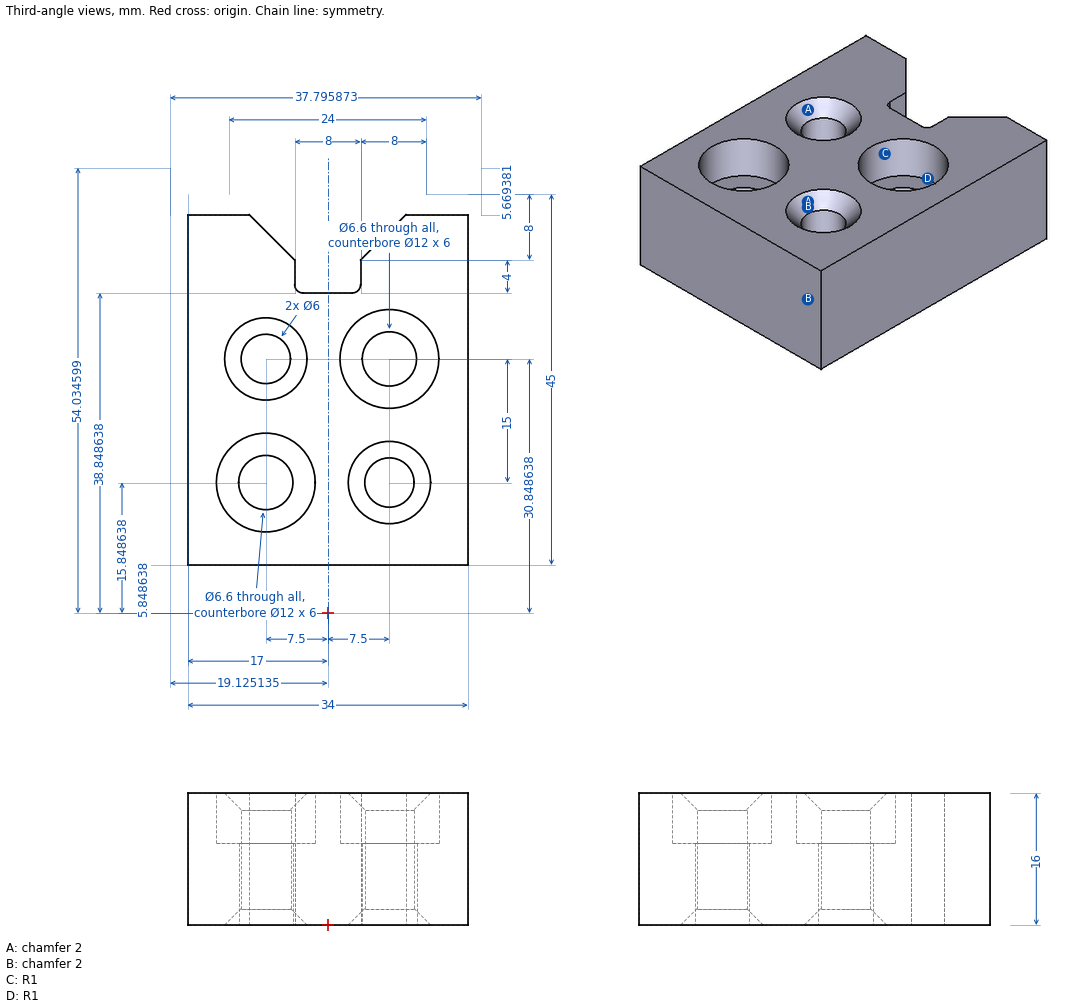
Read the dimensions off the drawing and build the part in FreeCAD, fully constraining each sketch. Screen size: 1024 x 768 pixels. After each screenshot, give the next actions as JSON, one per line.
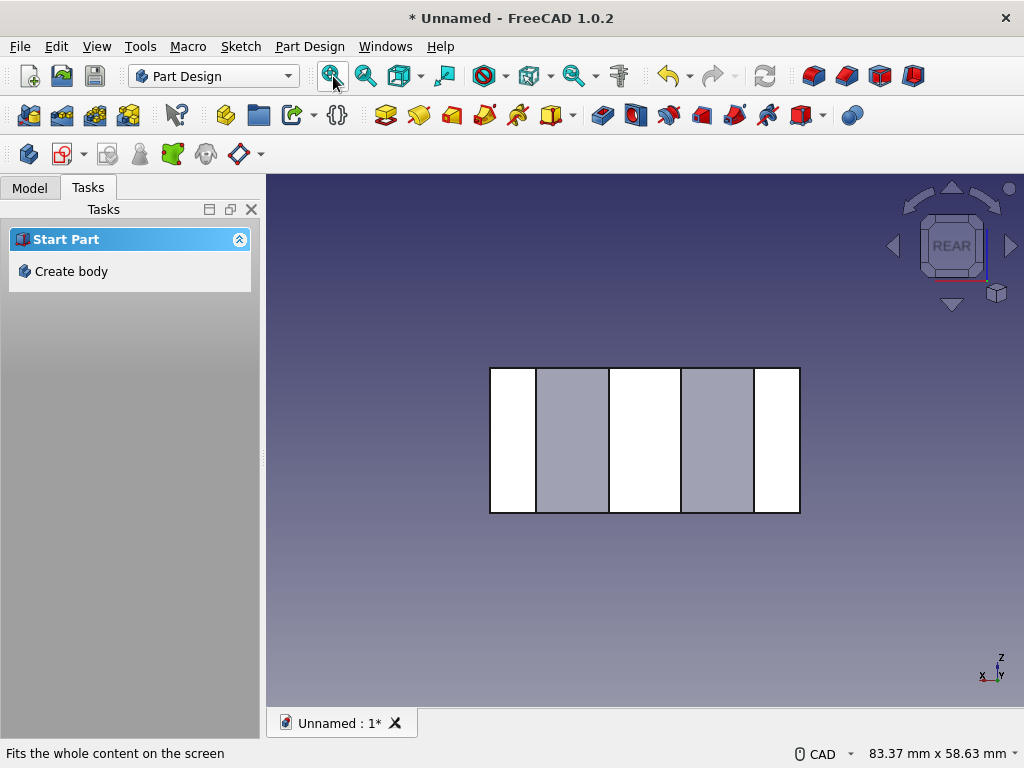
{"action": "left_click", "coordinate": [333, 76]}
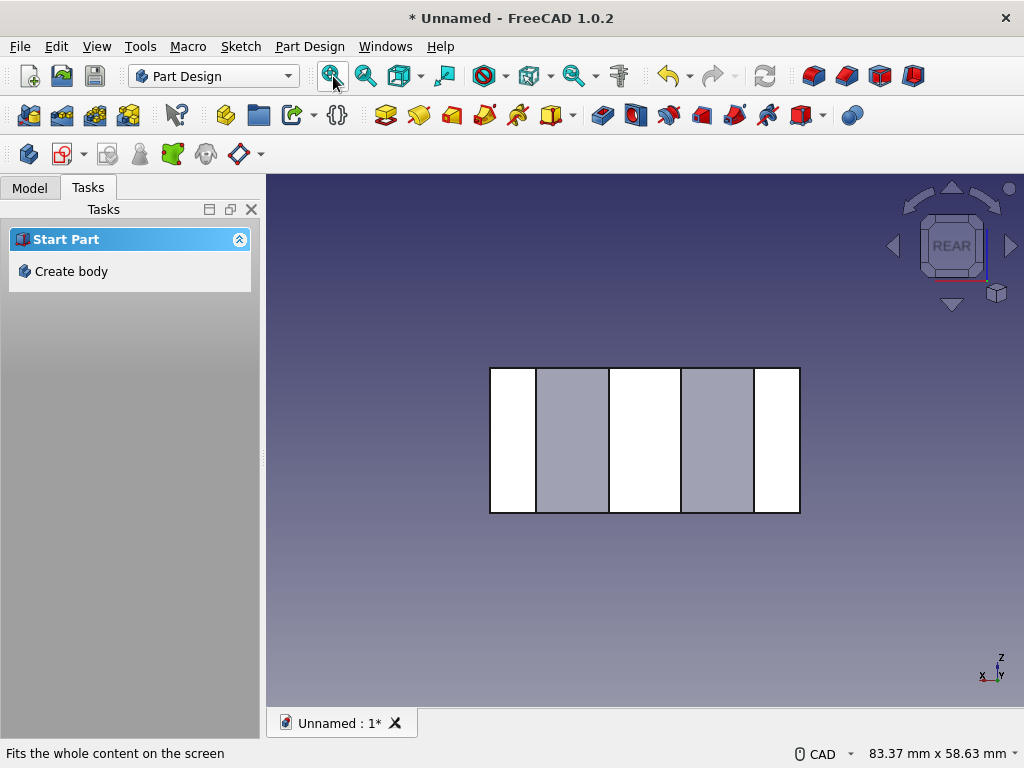
{"action": "key", "text": "6"}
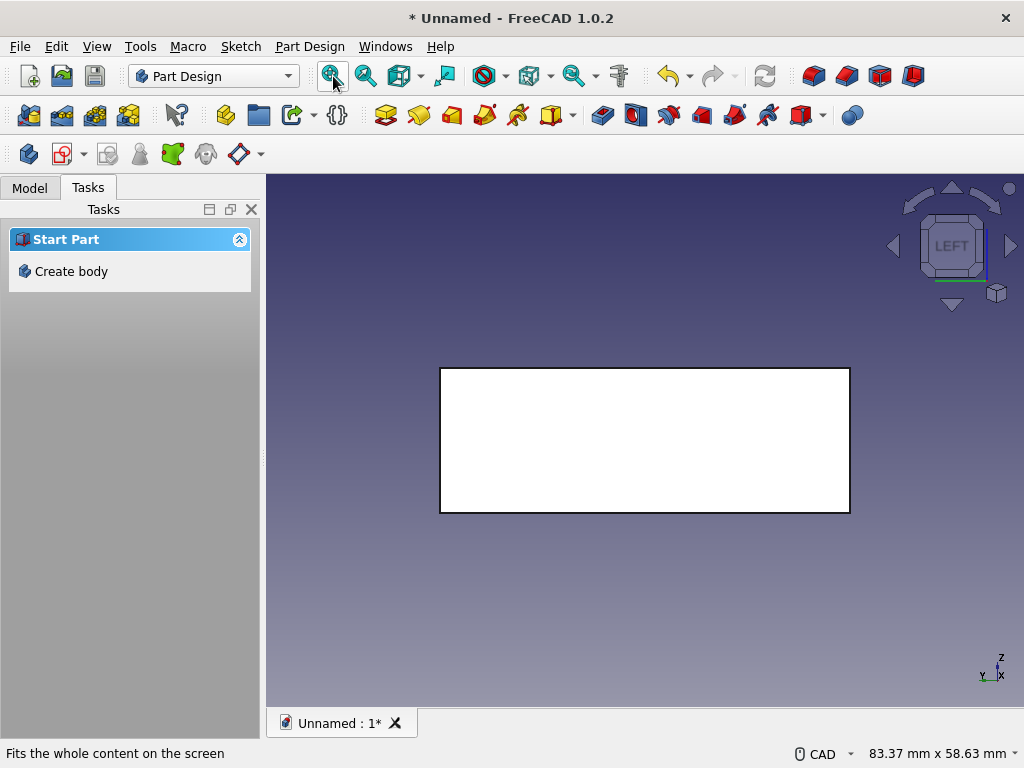
{"action": "key", "text": "v 3"}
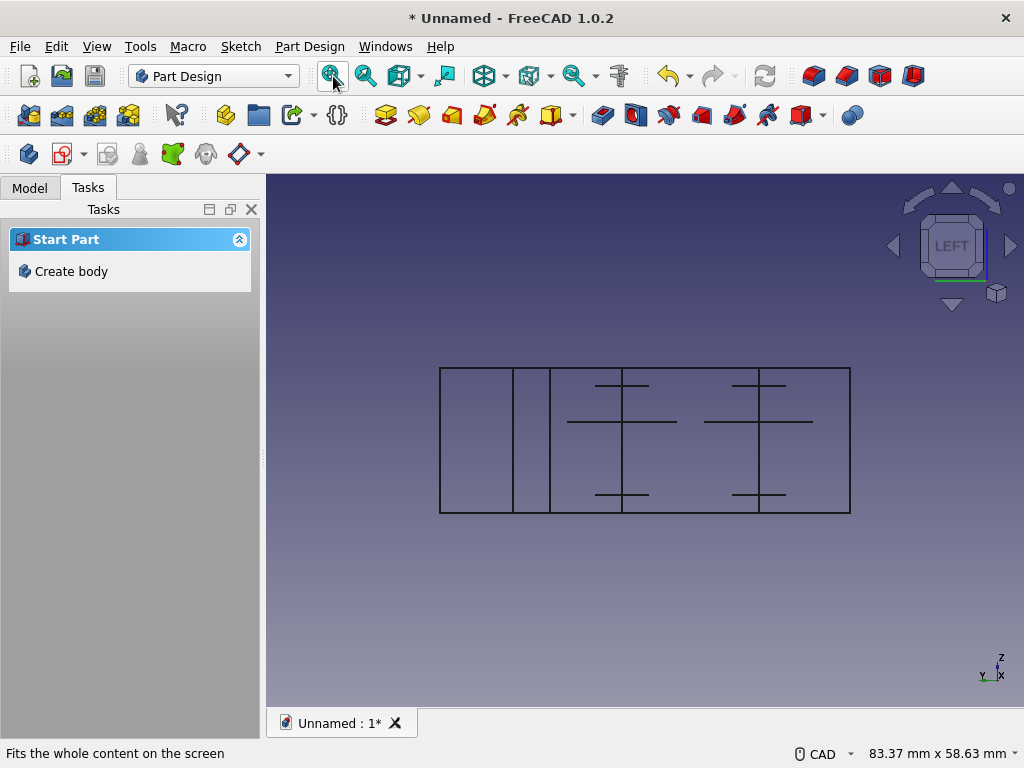
{"action": "key", "text": "0"}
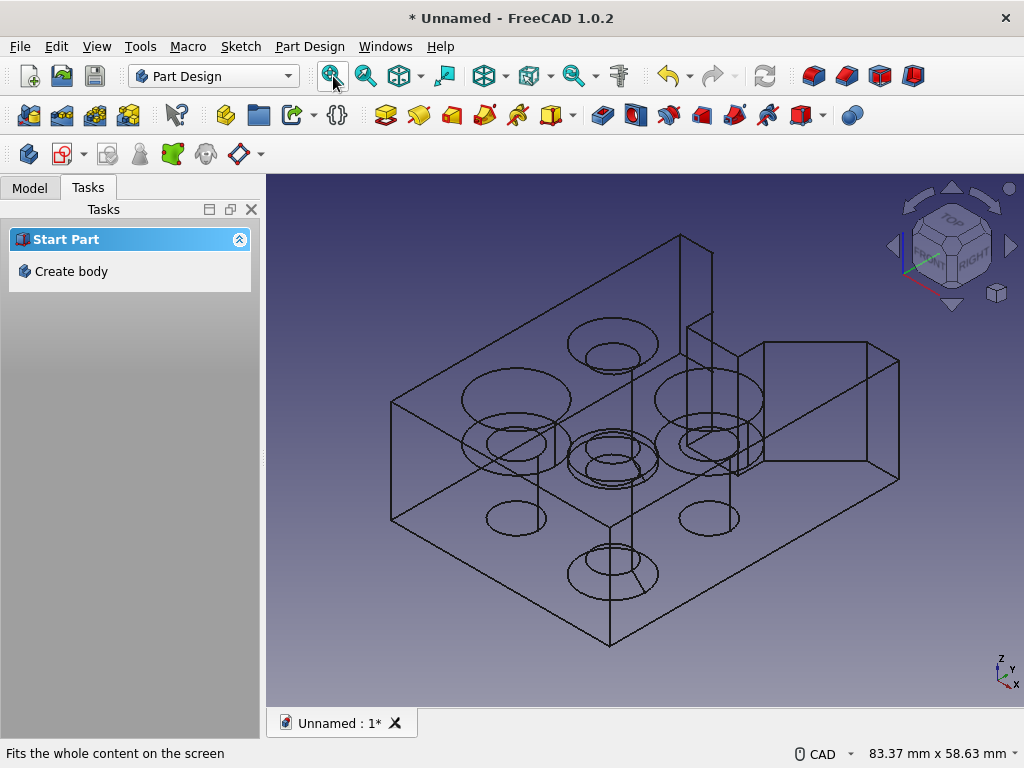
{"action": "left_click", "coordinate": [687, 386]}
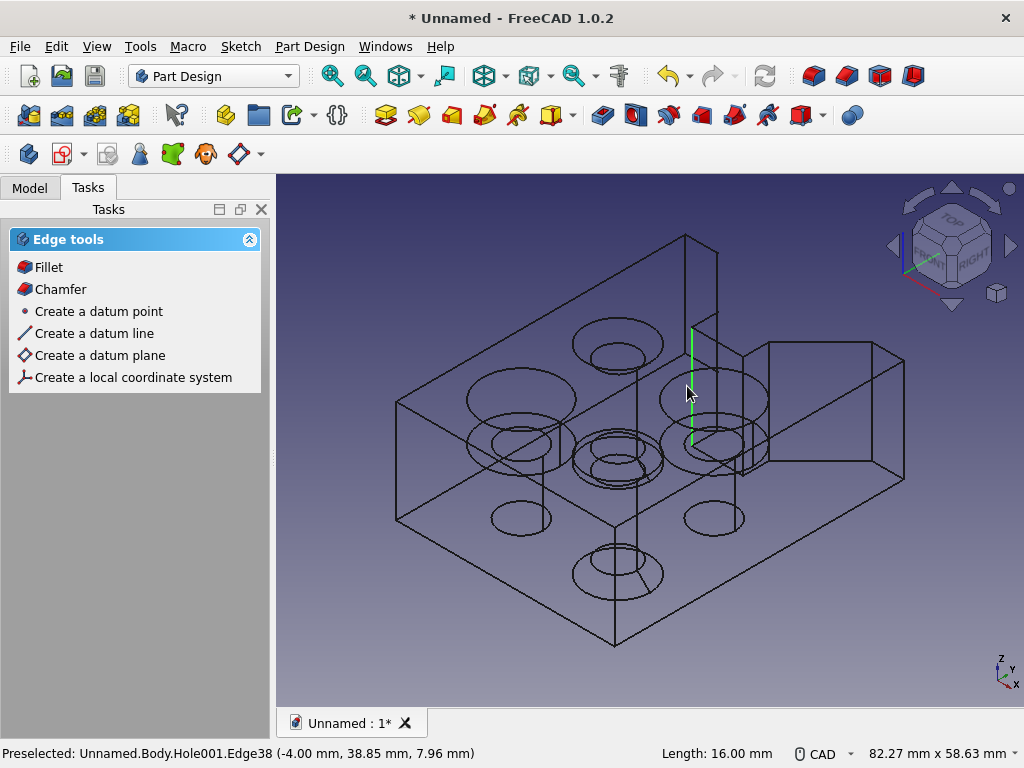
{"action": "key", "text": "v 1"}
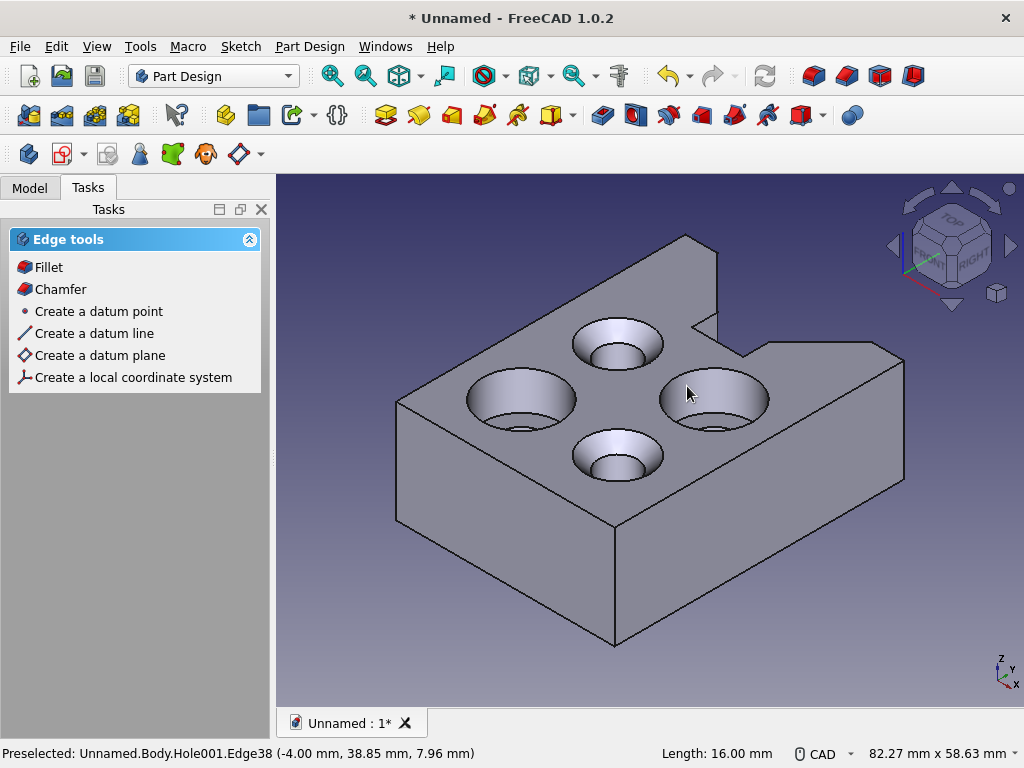
{"action": "left_click", "coordinate": [814, 76]}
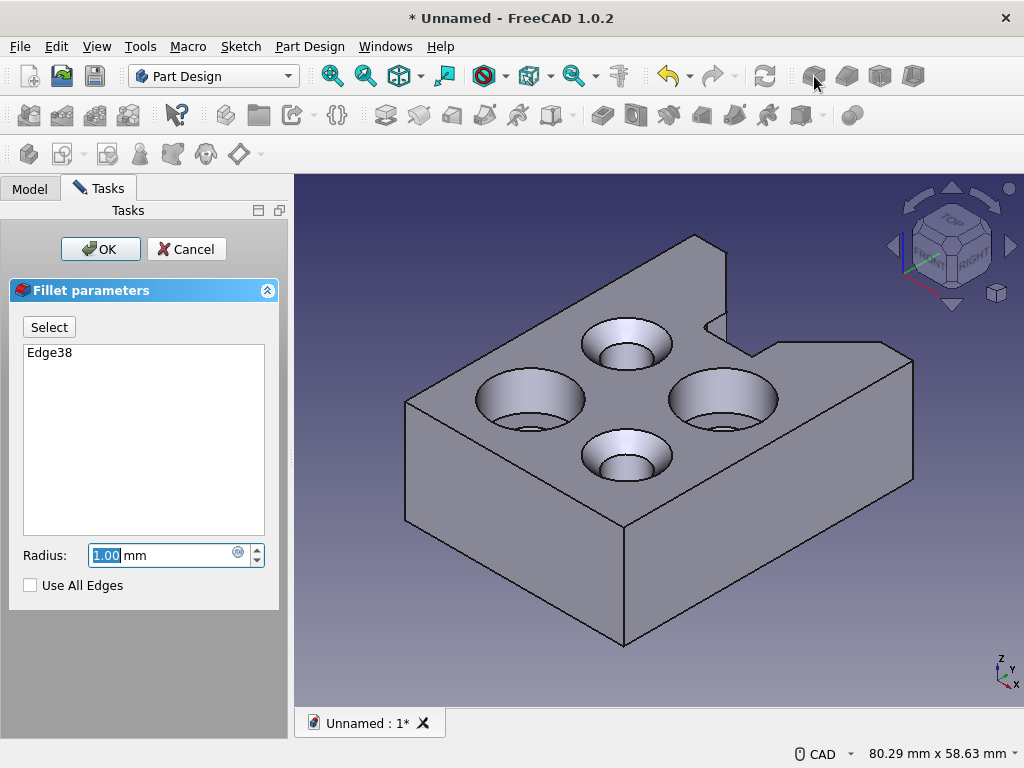
{"action": "type", "text": "1"}
{"action": "key", "text": "Tab"}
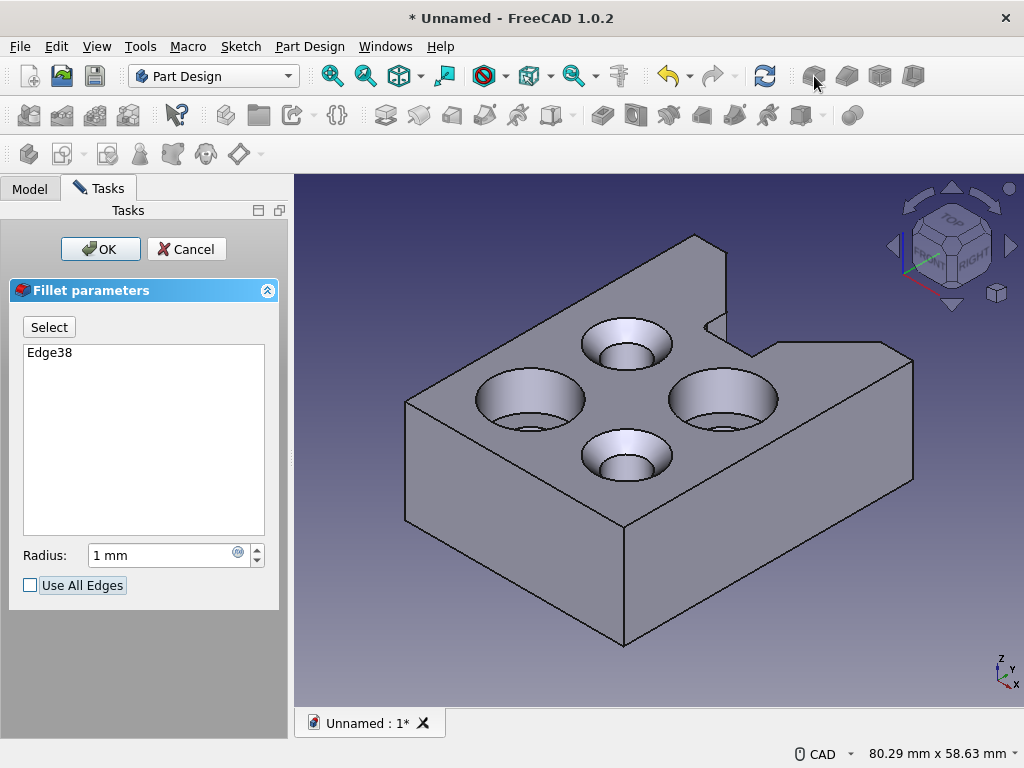
{"action": "left_click", "coordinate": [101, 249]}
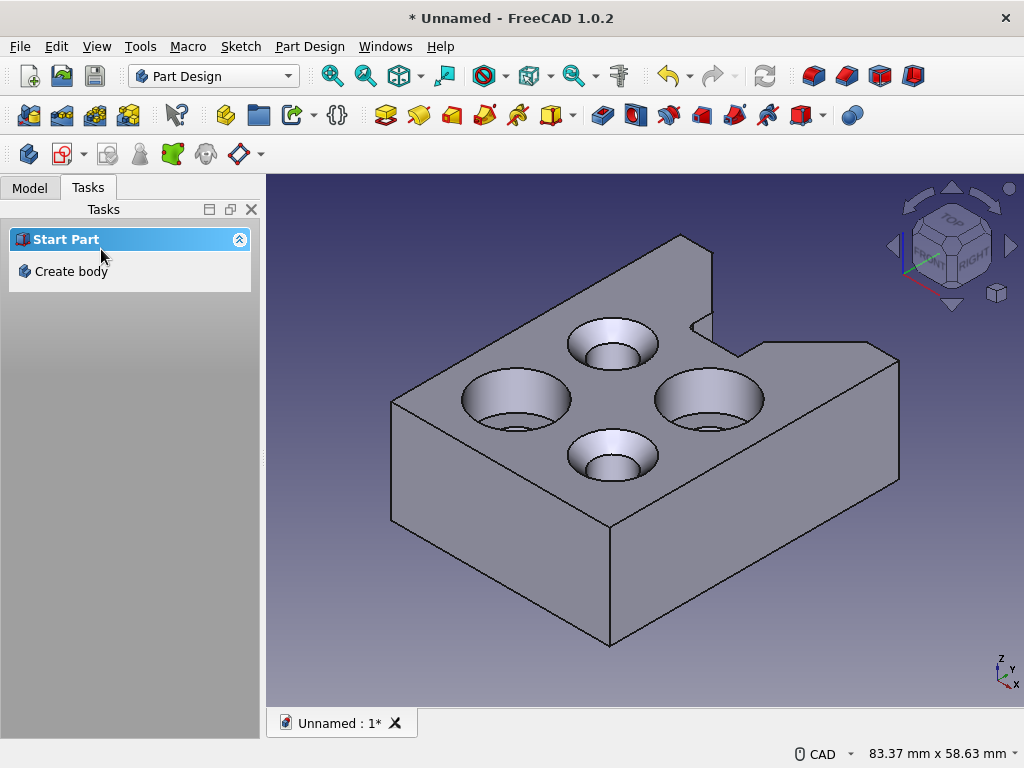
{"action": "key", "text": "2"}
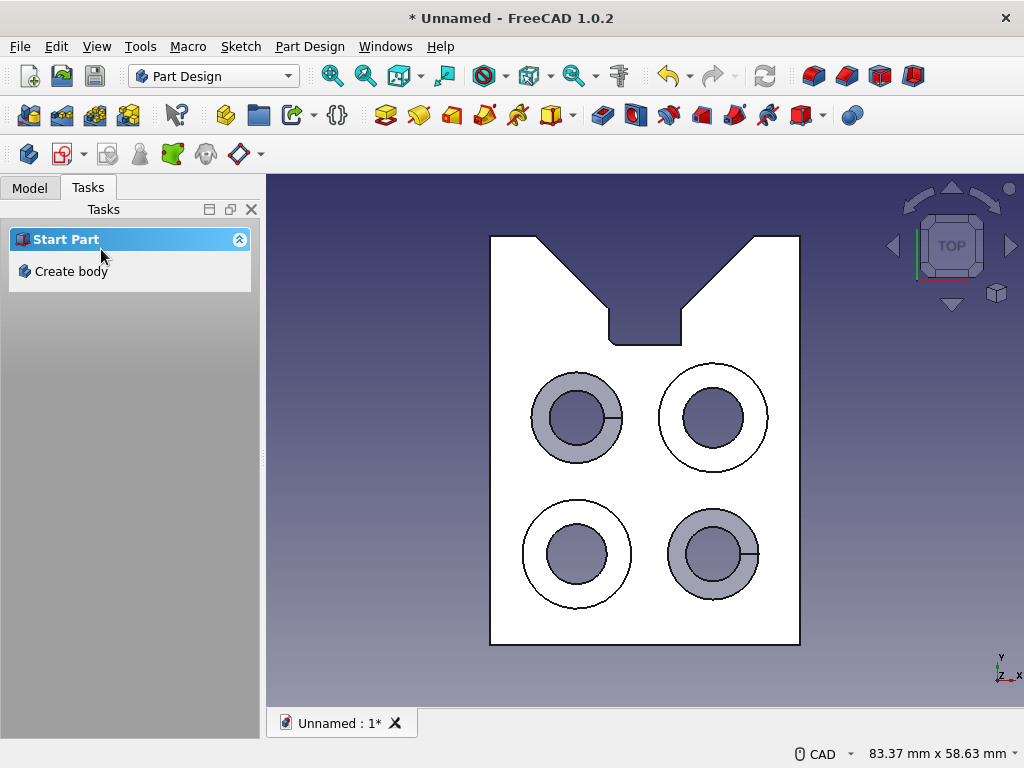
{"action": "key", "text": "0"}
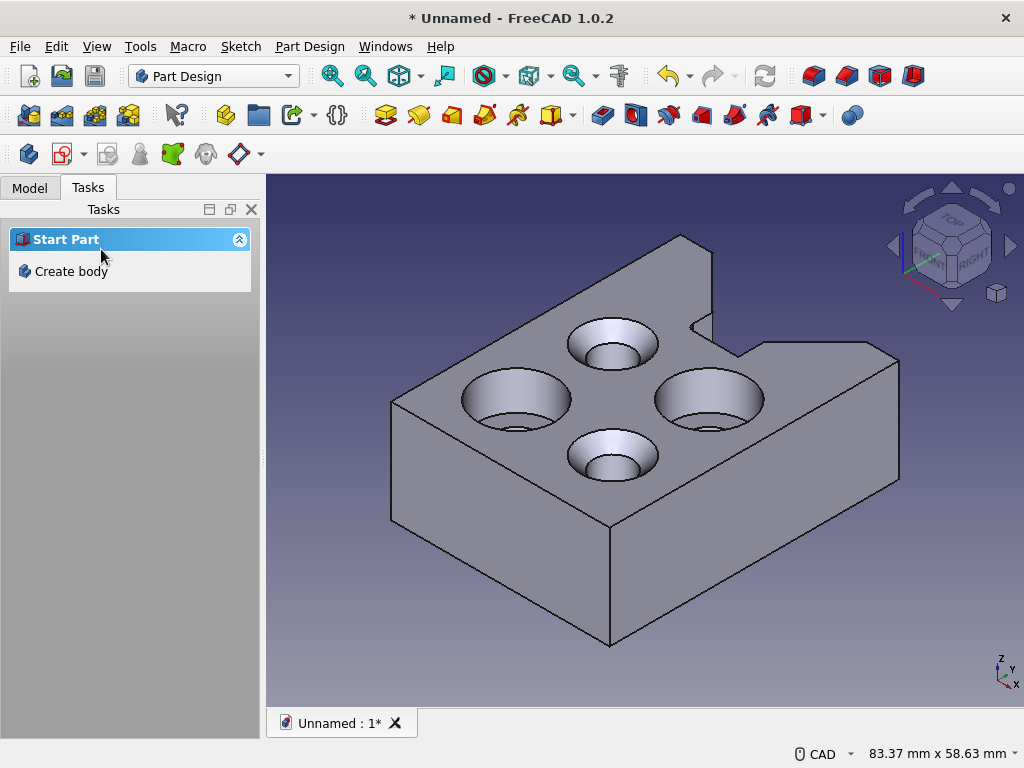
{"action": "key", "text": "1"}